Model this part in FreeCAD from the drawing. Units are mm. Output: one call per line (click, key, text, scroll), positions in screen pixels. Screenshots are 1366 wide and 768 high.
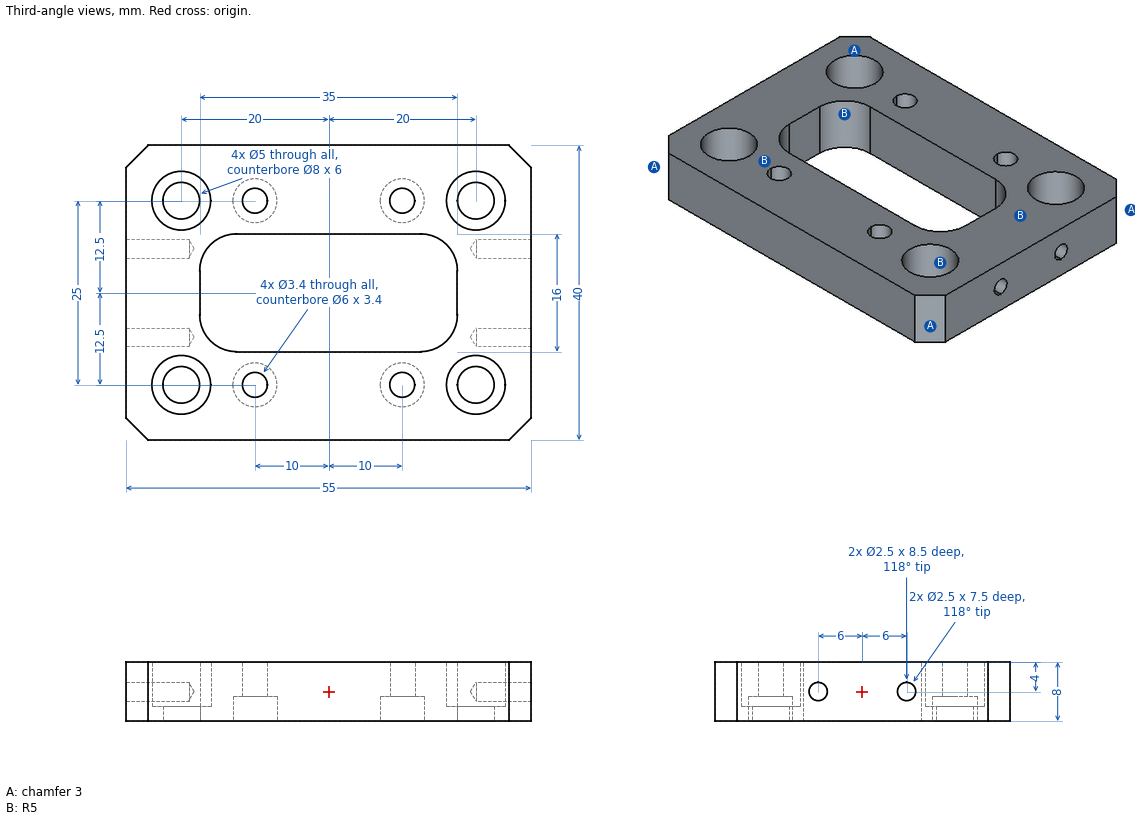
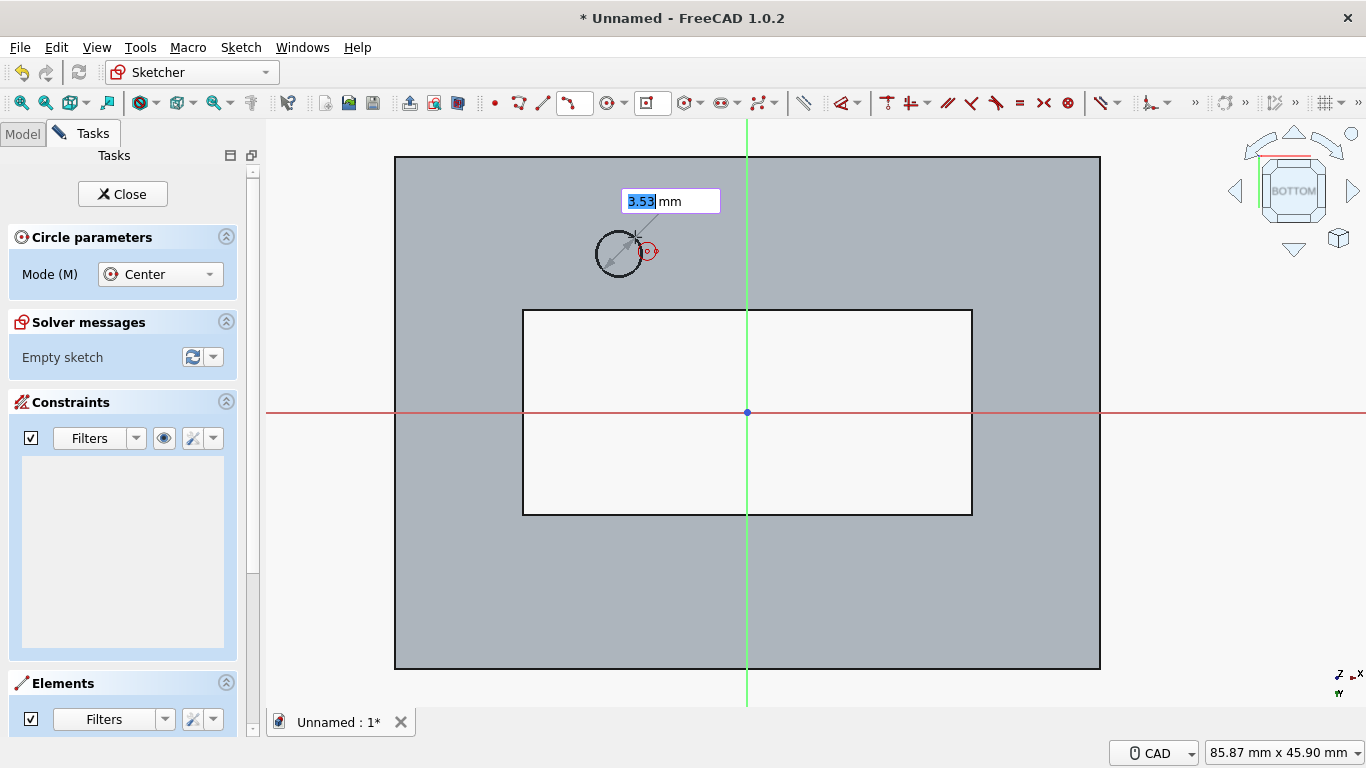
text(3.4)
key(Return)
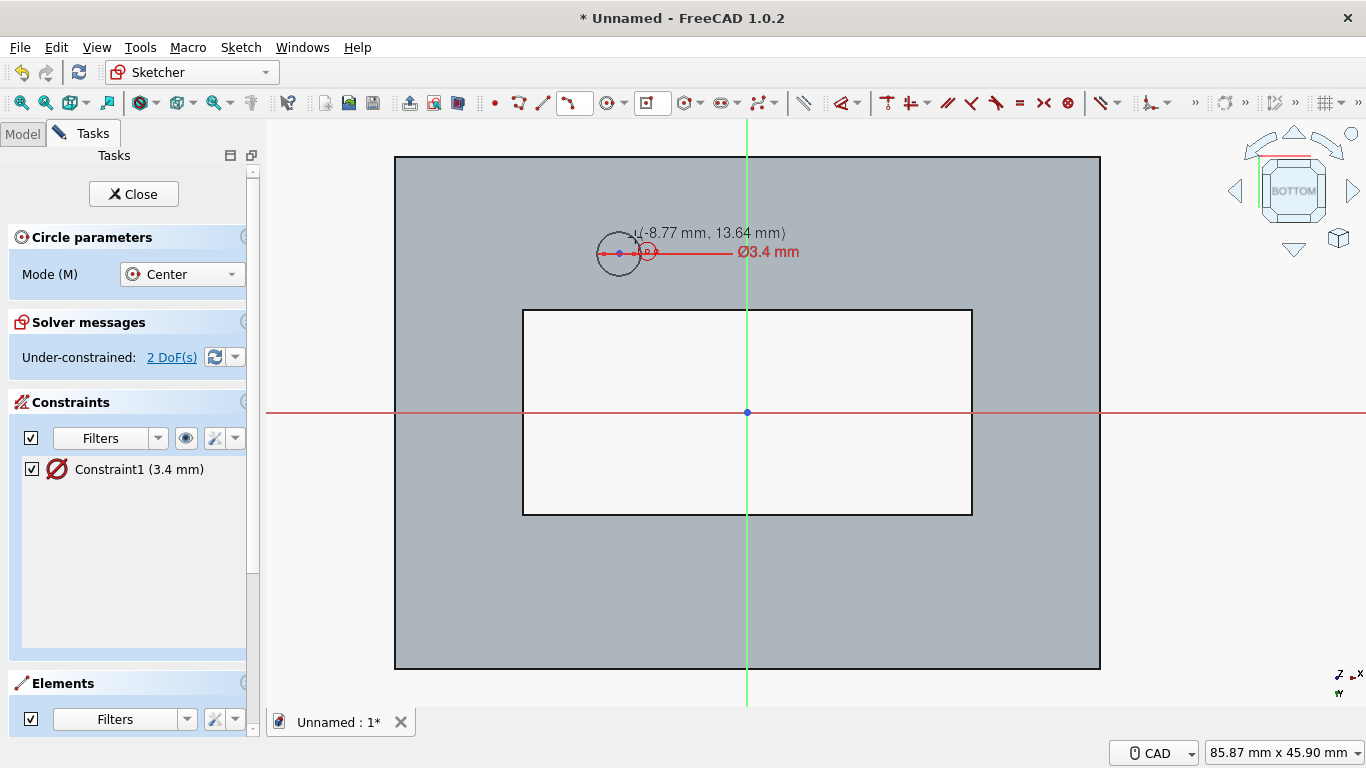
click(875, 253)
move(891, 237)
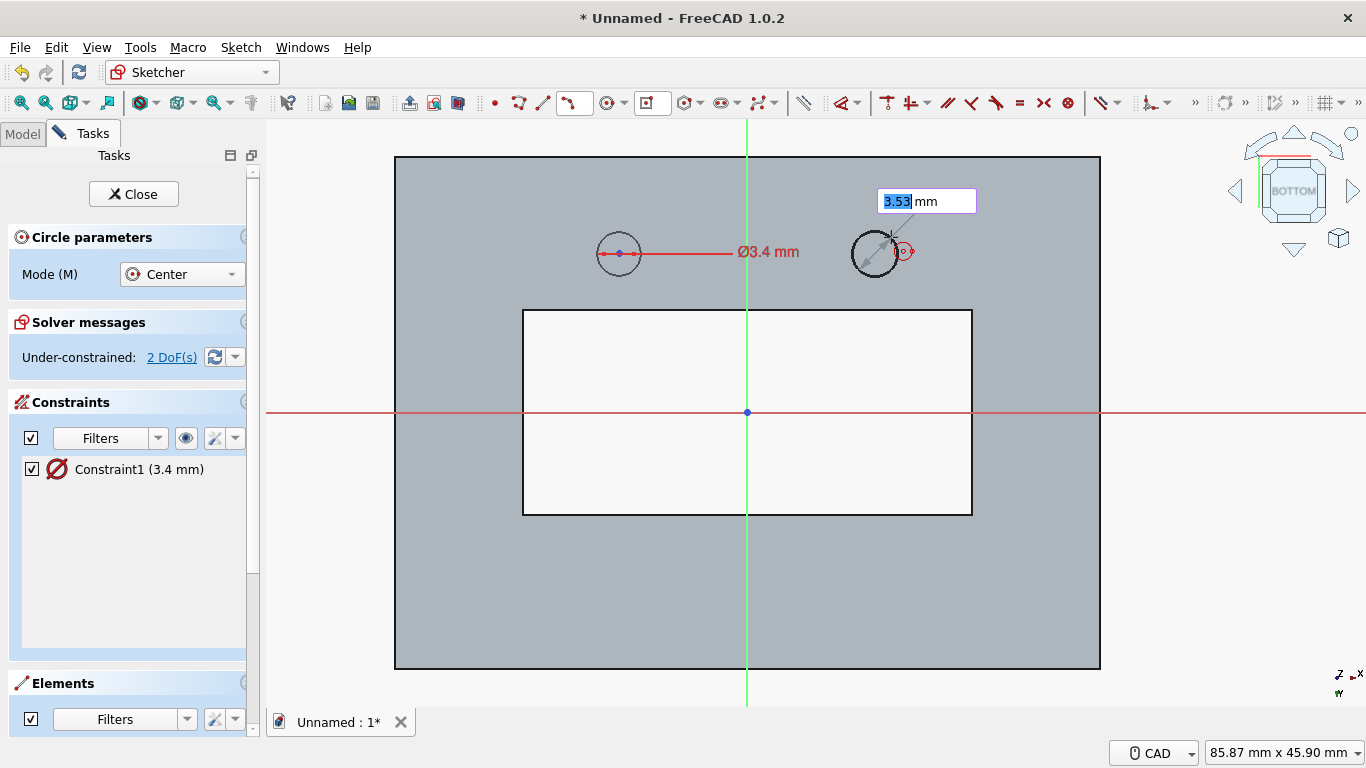
text(3.4)
key(Return)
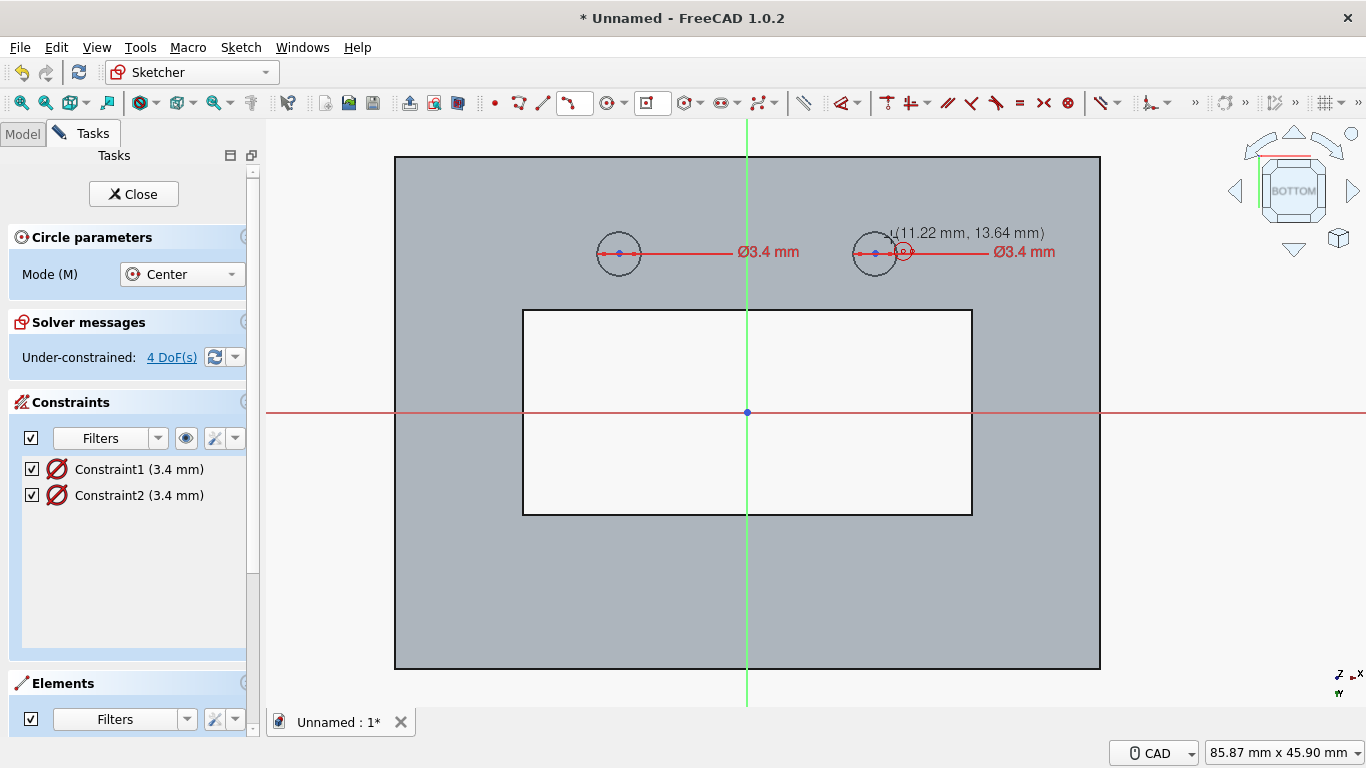
click(619, 573)
move(635, 557)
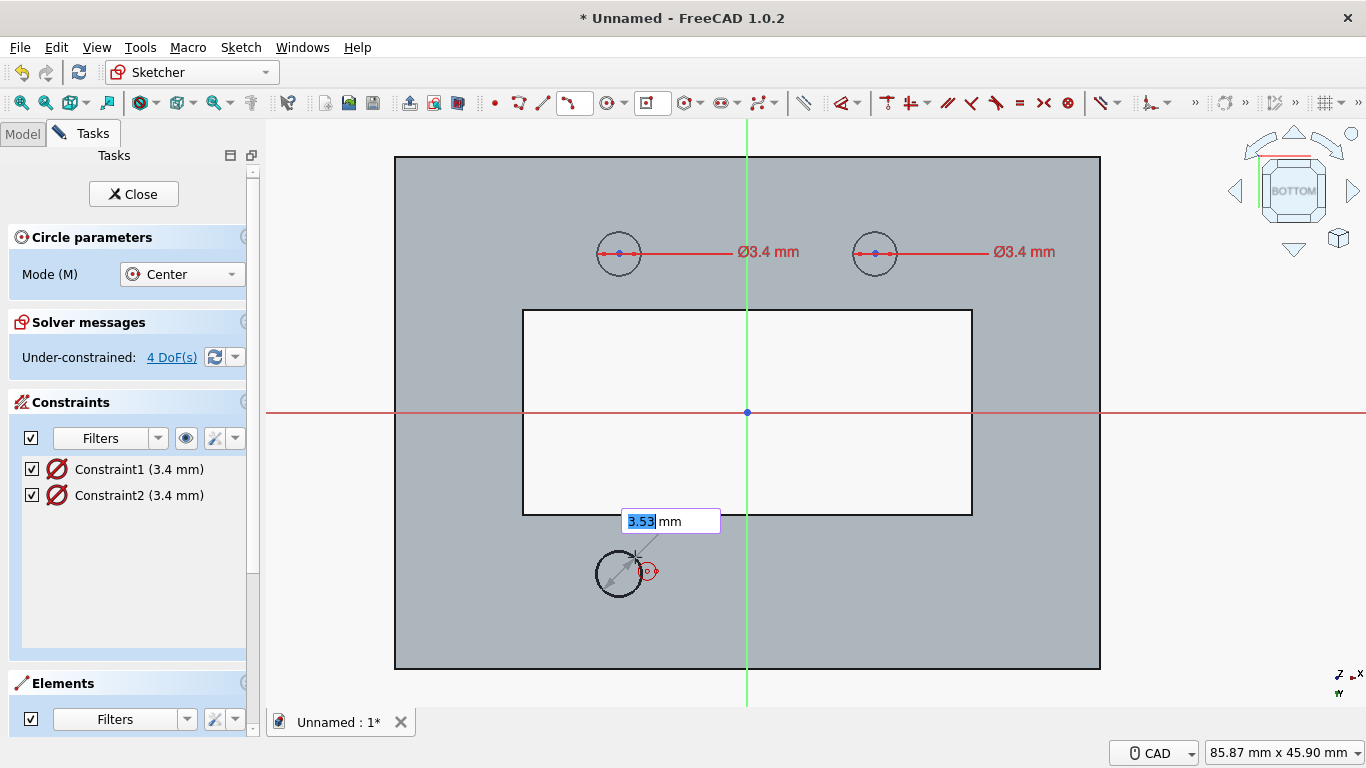
text(3.4)
key(Return)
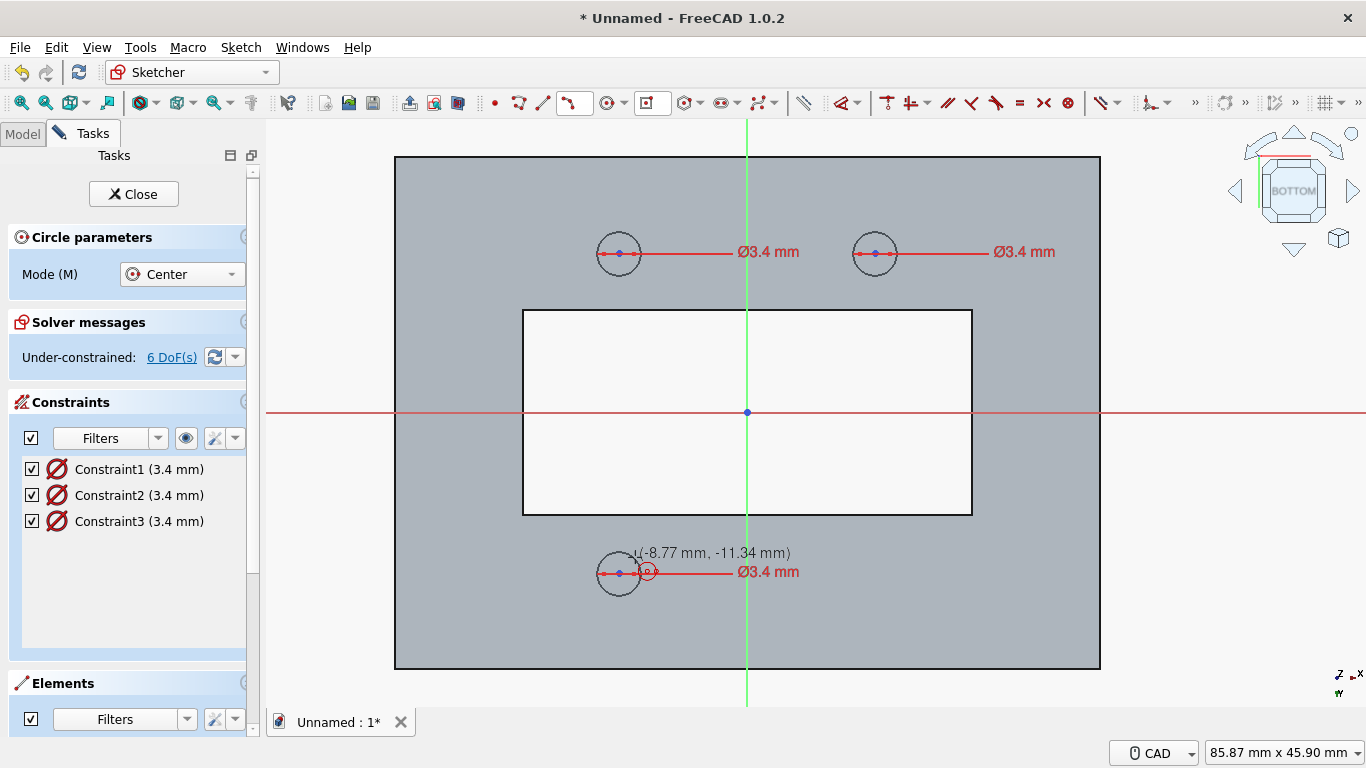
click(875, 573)
move(891, 557)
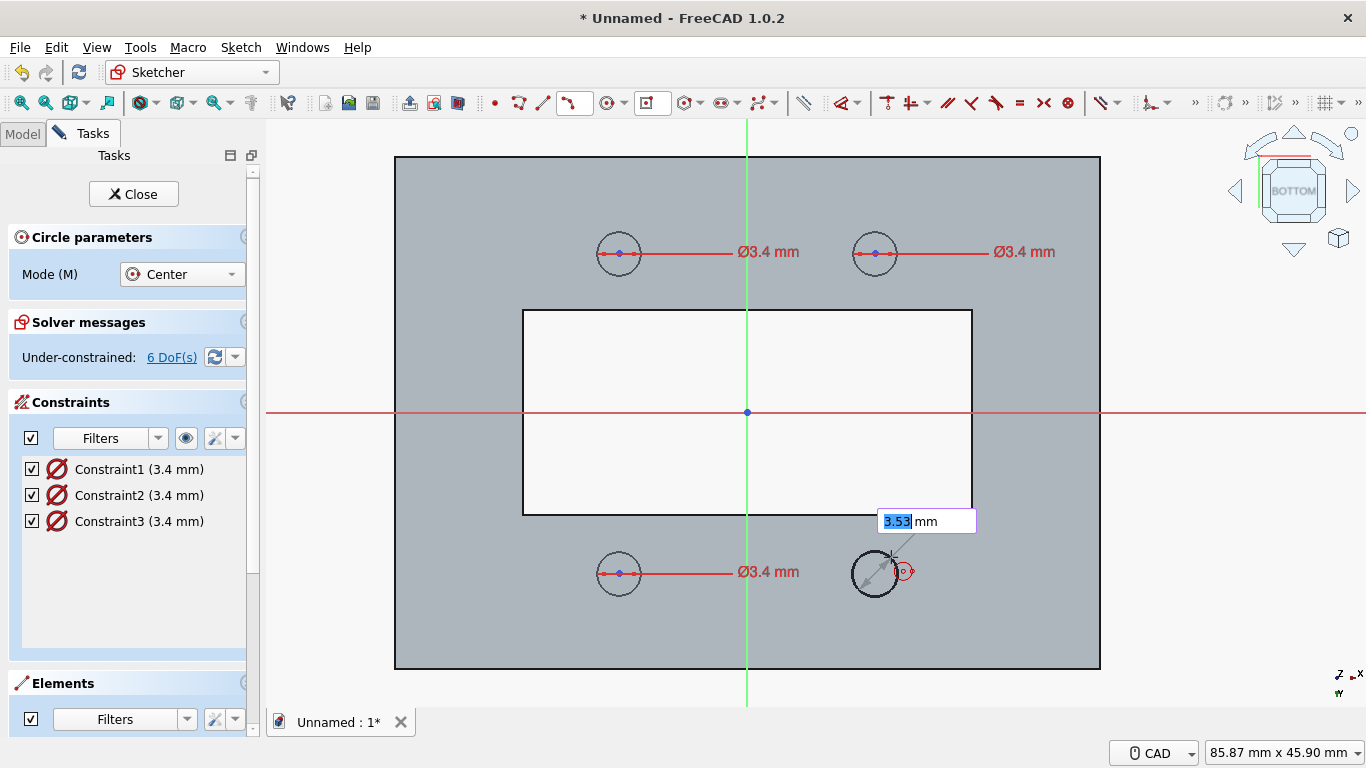
text(3.4)
key(Return)
key(Escape)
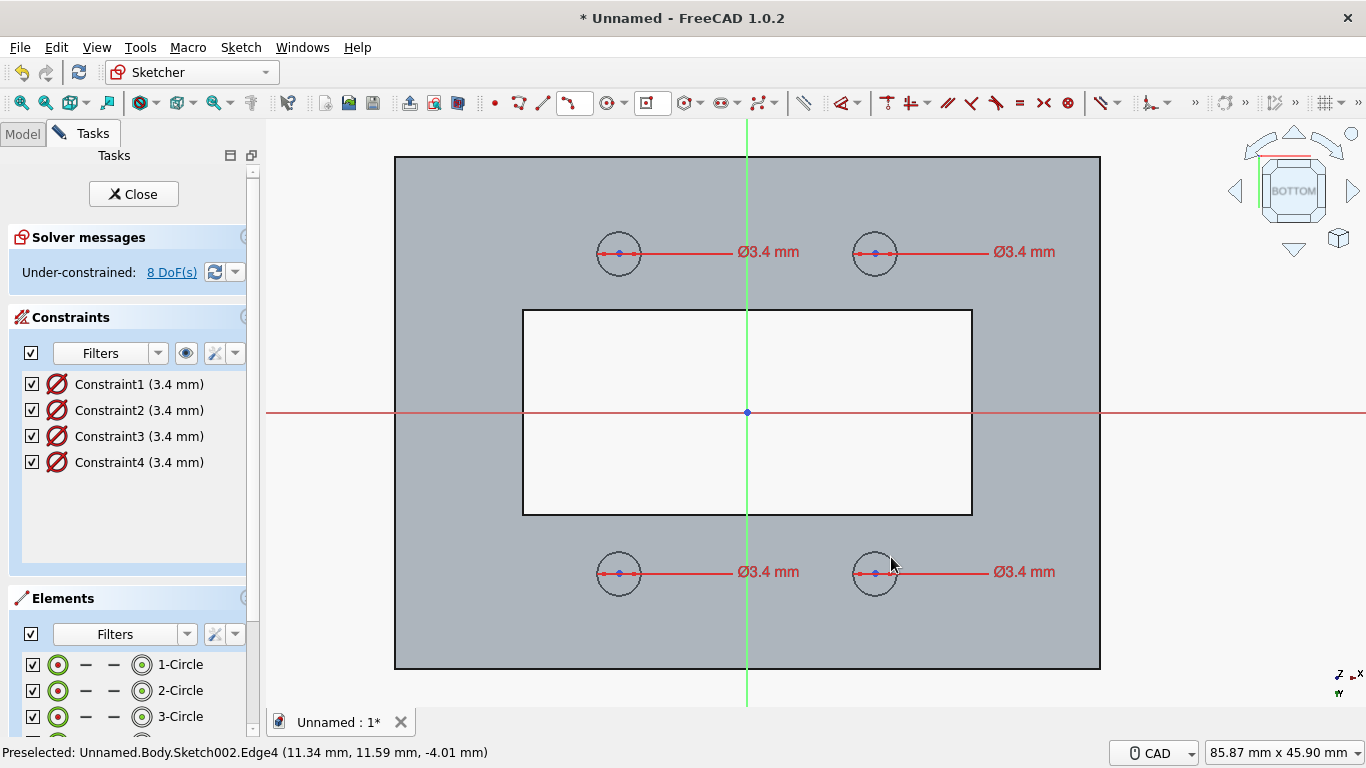
click(619, 254)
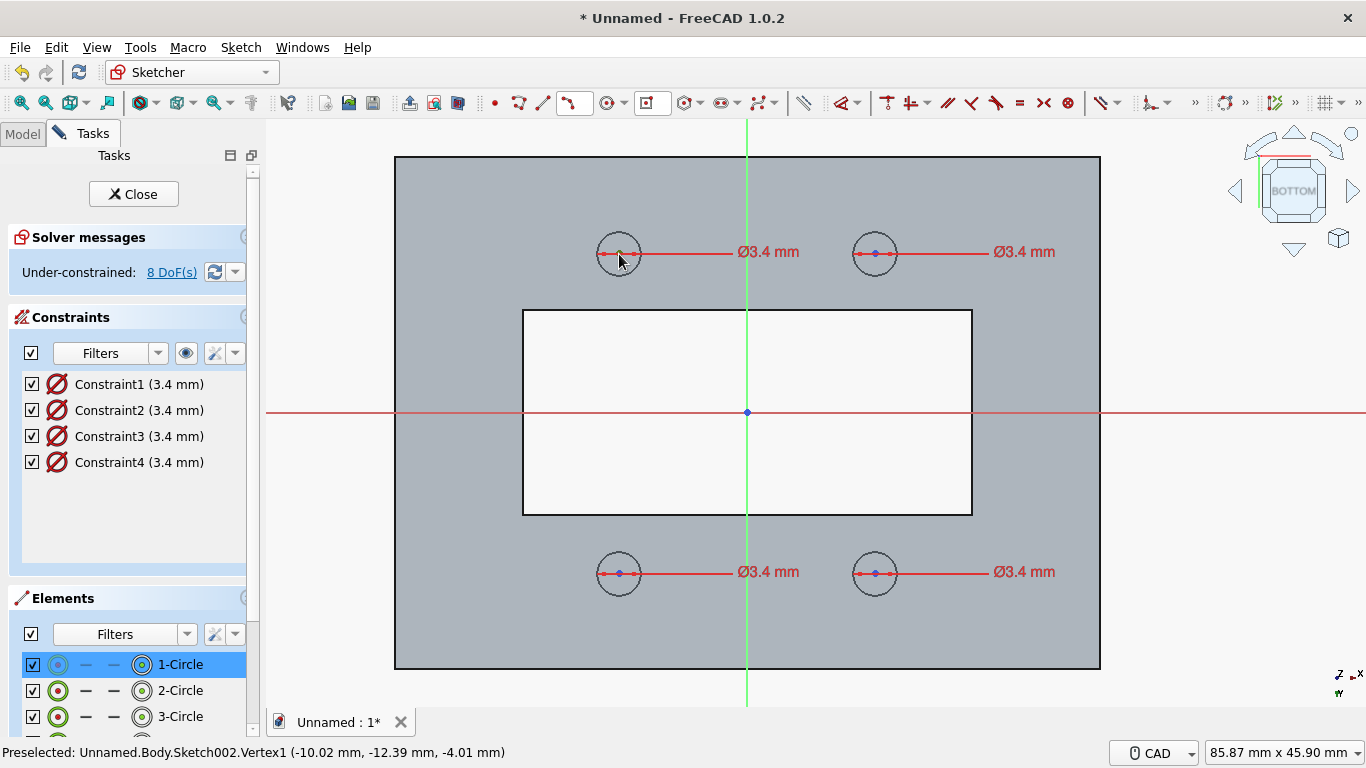
click(875, 254)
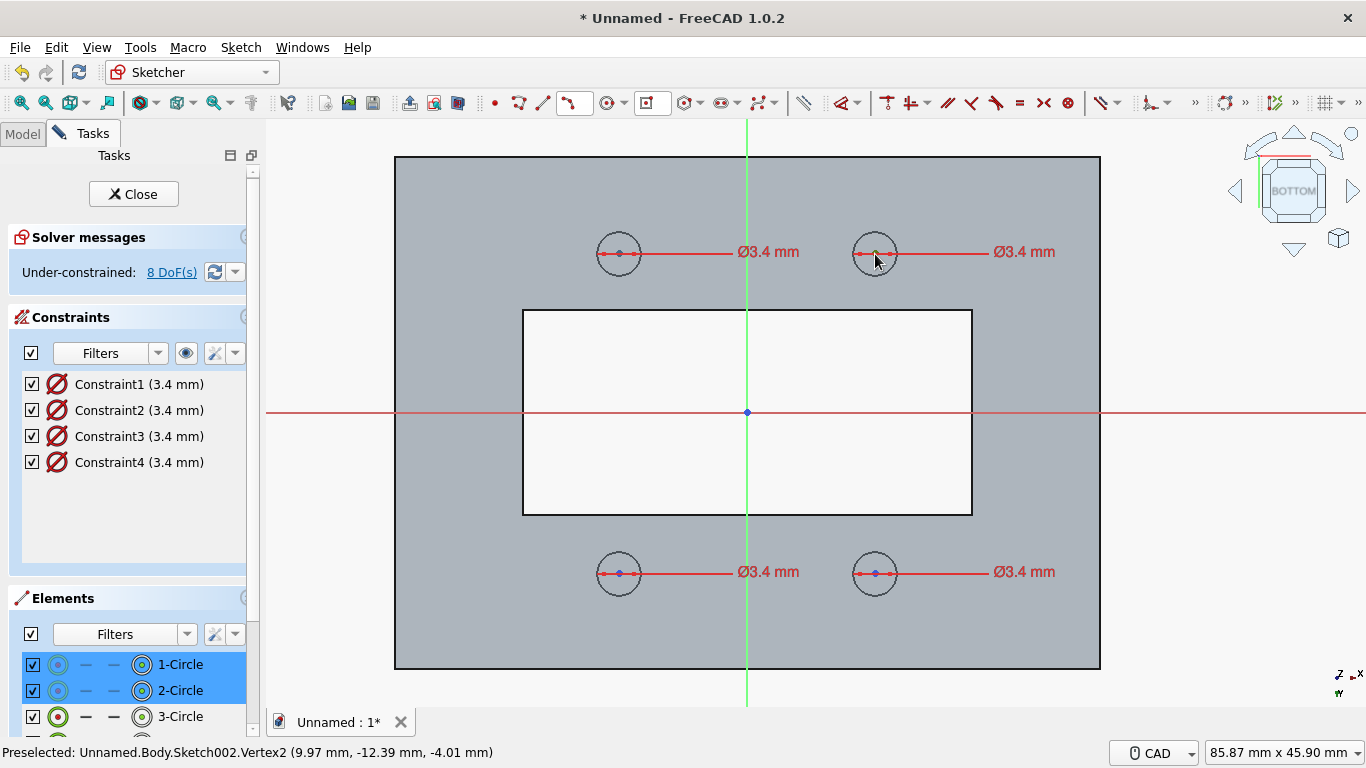
key(h)